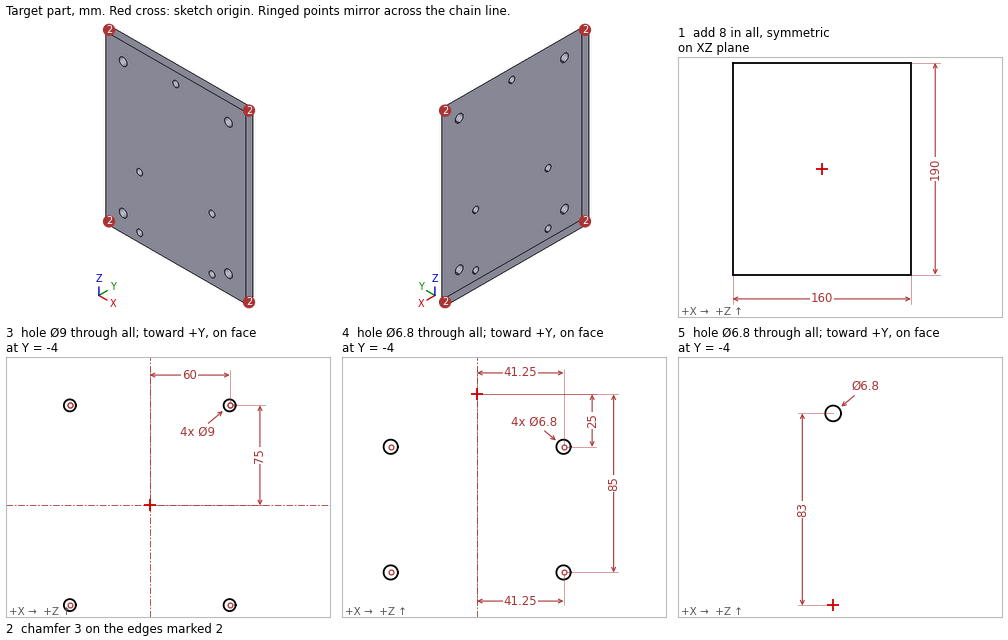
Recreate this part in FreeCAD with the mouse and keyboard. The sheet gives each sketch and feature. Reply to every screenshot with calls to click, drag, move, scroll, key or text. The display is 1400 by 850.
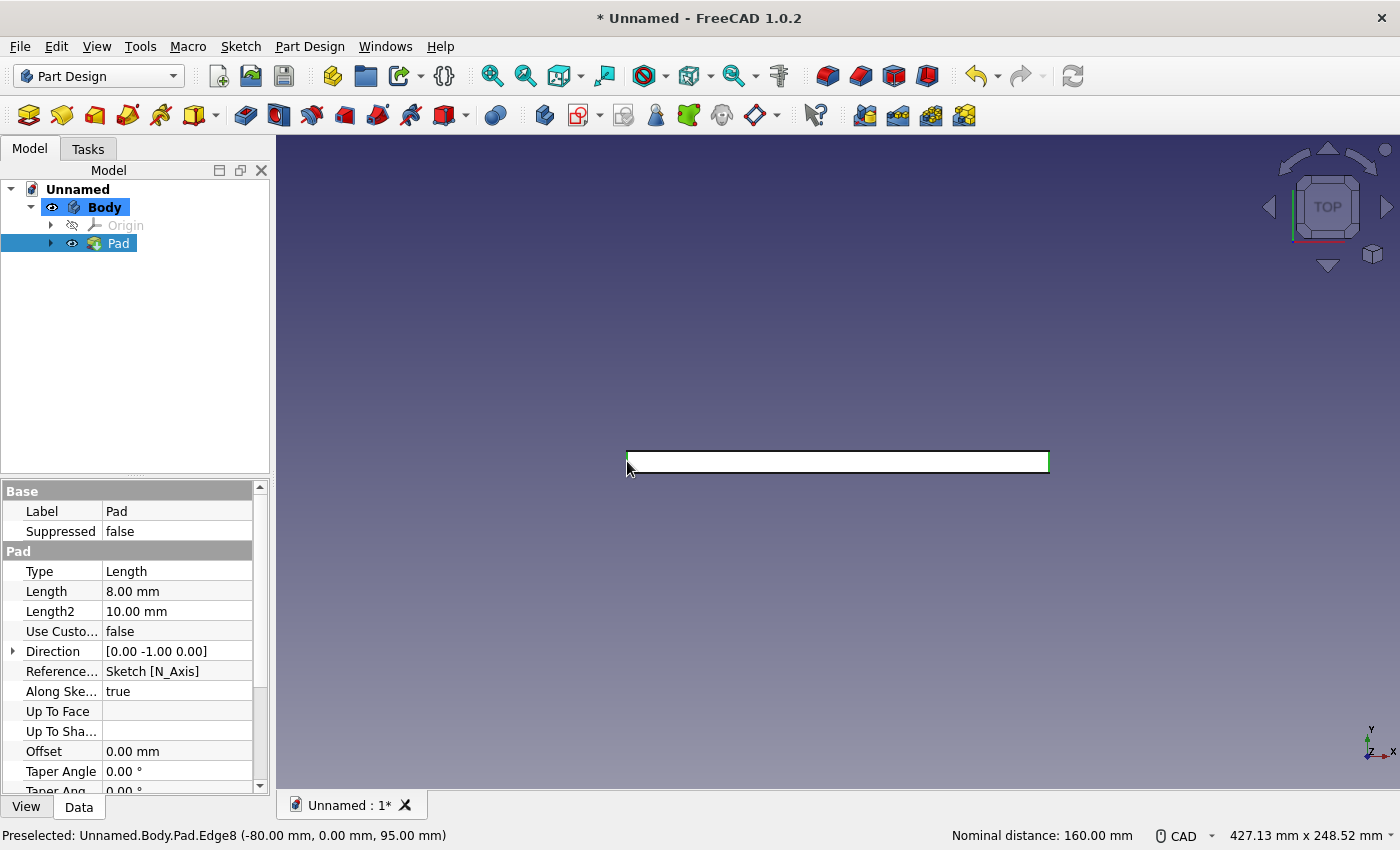
scroll(627, 461, up, 4)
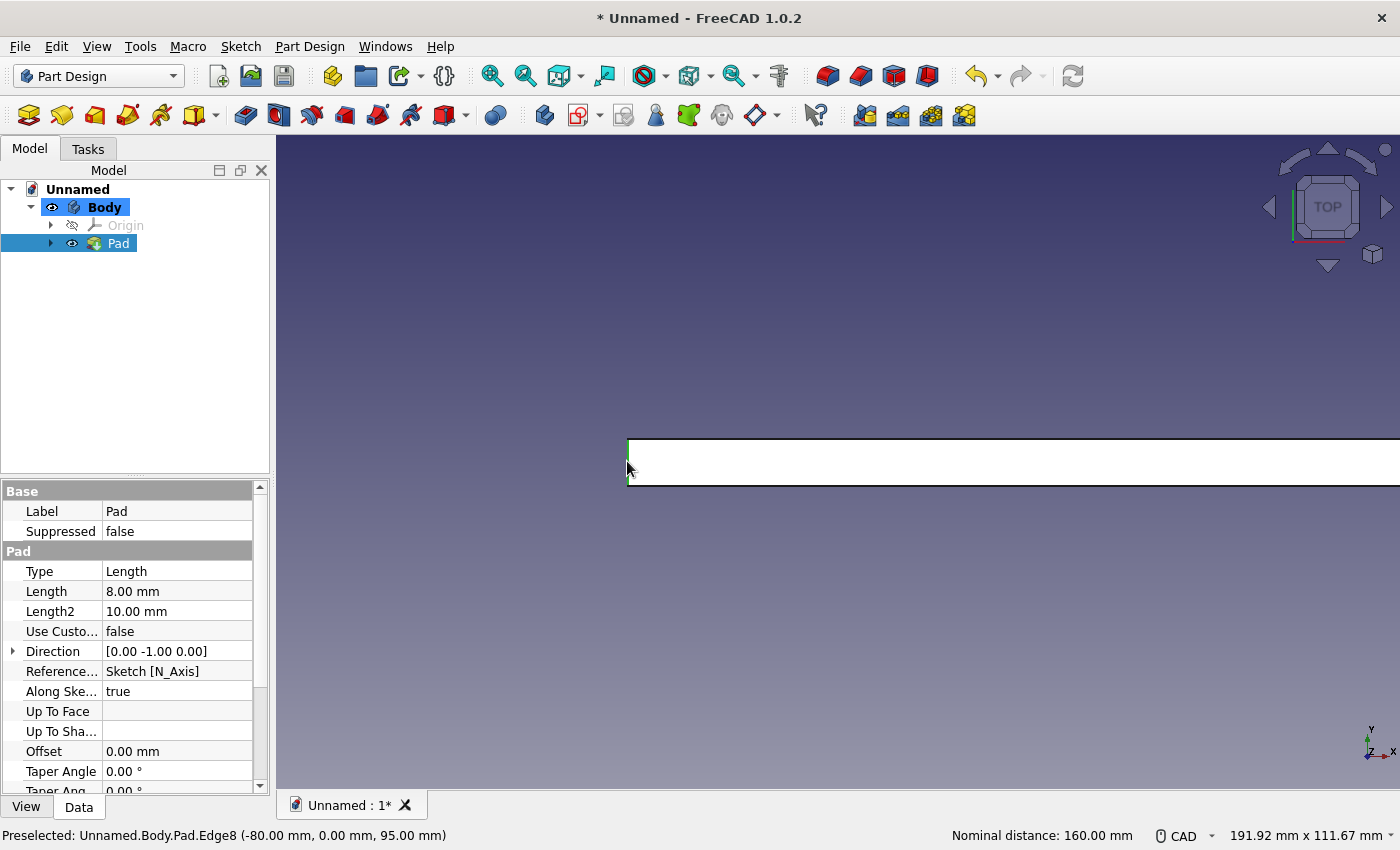
key(v)
key(f)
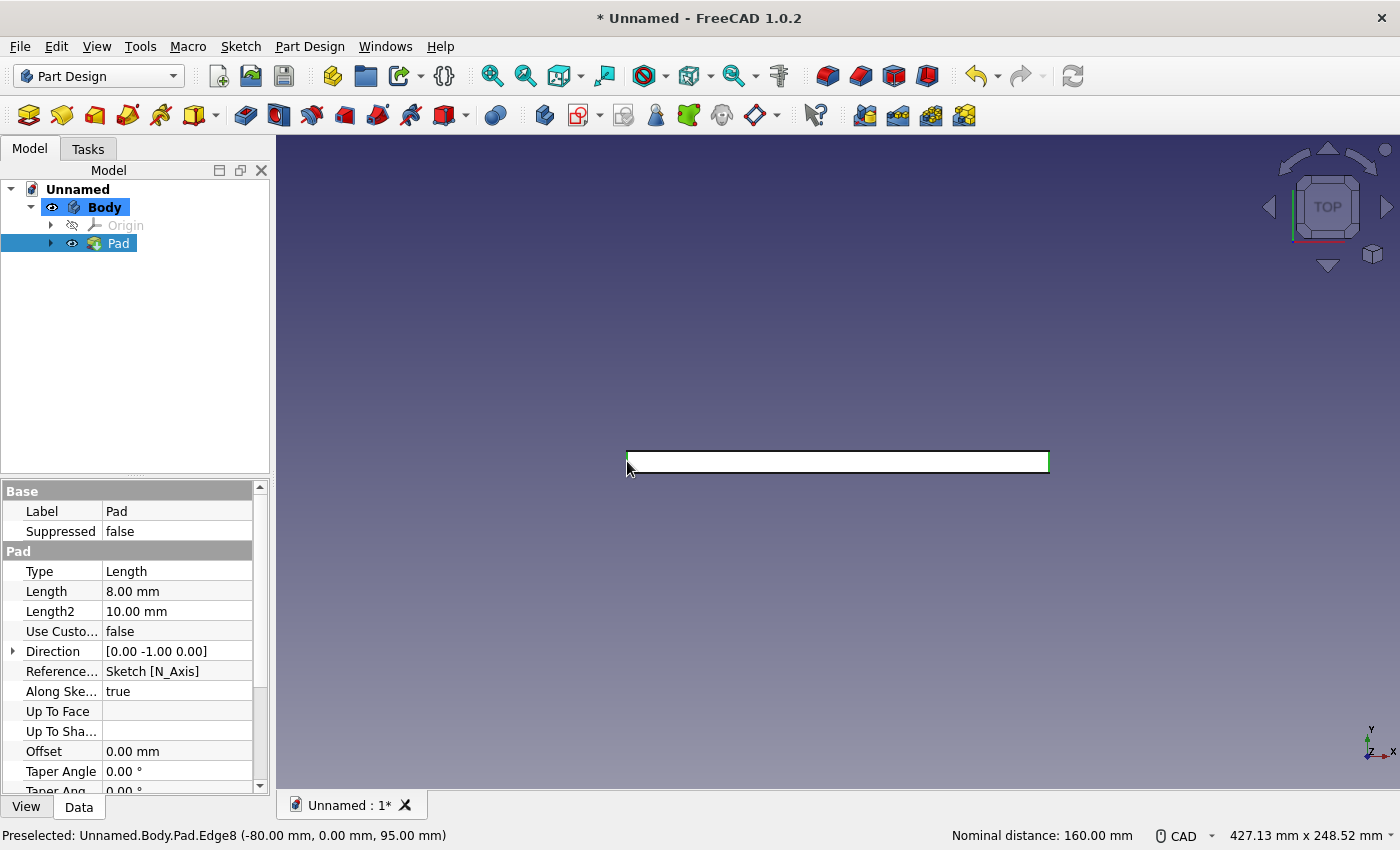
key(1)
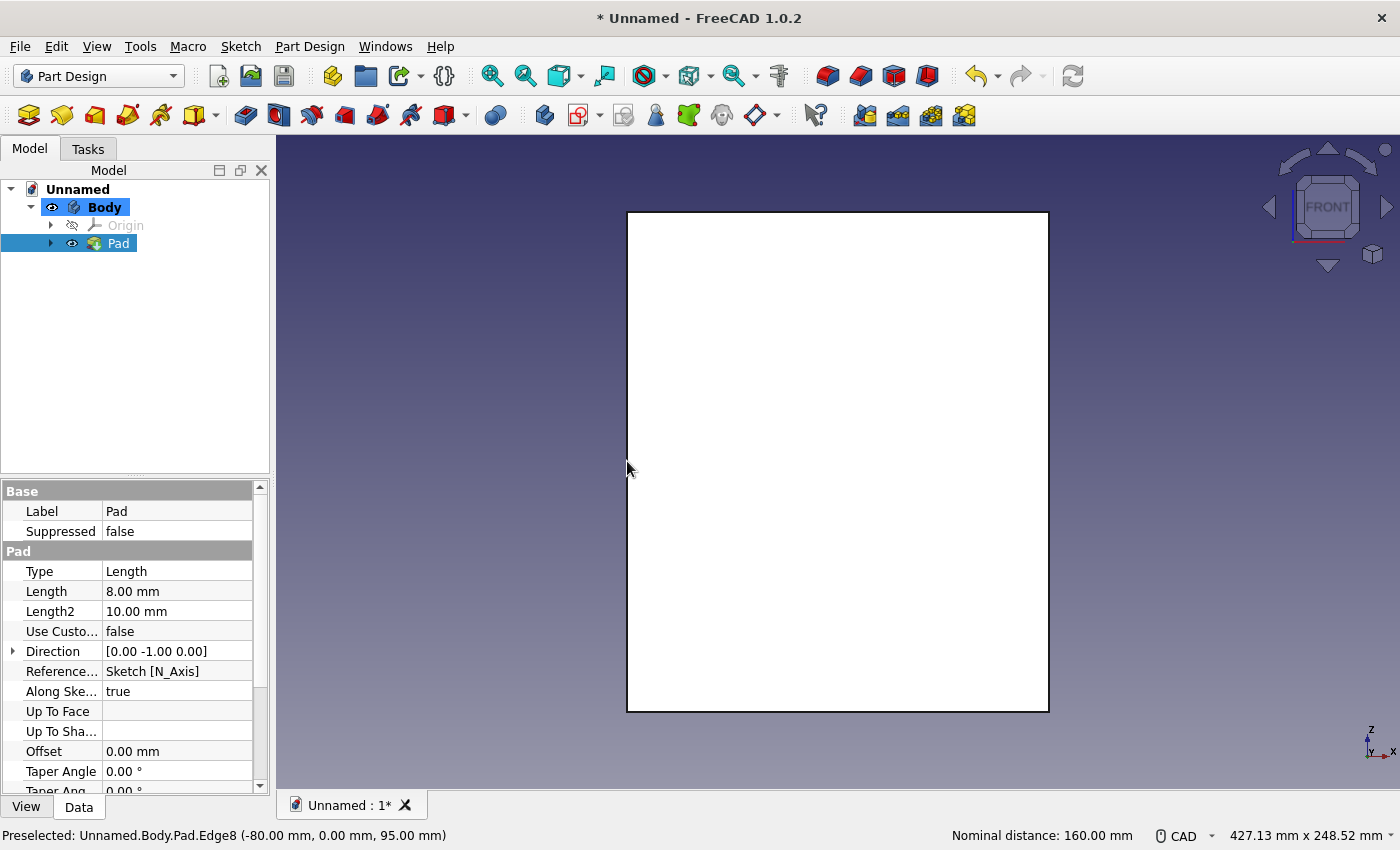
scroll(627, 711, up, 4)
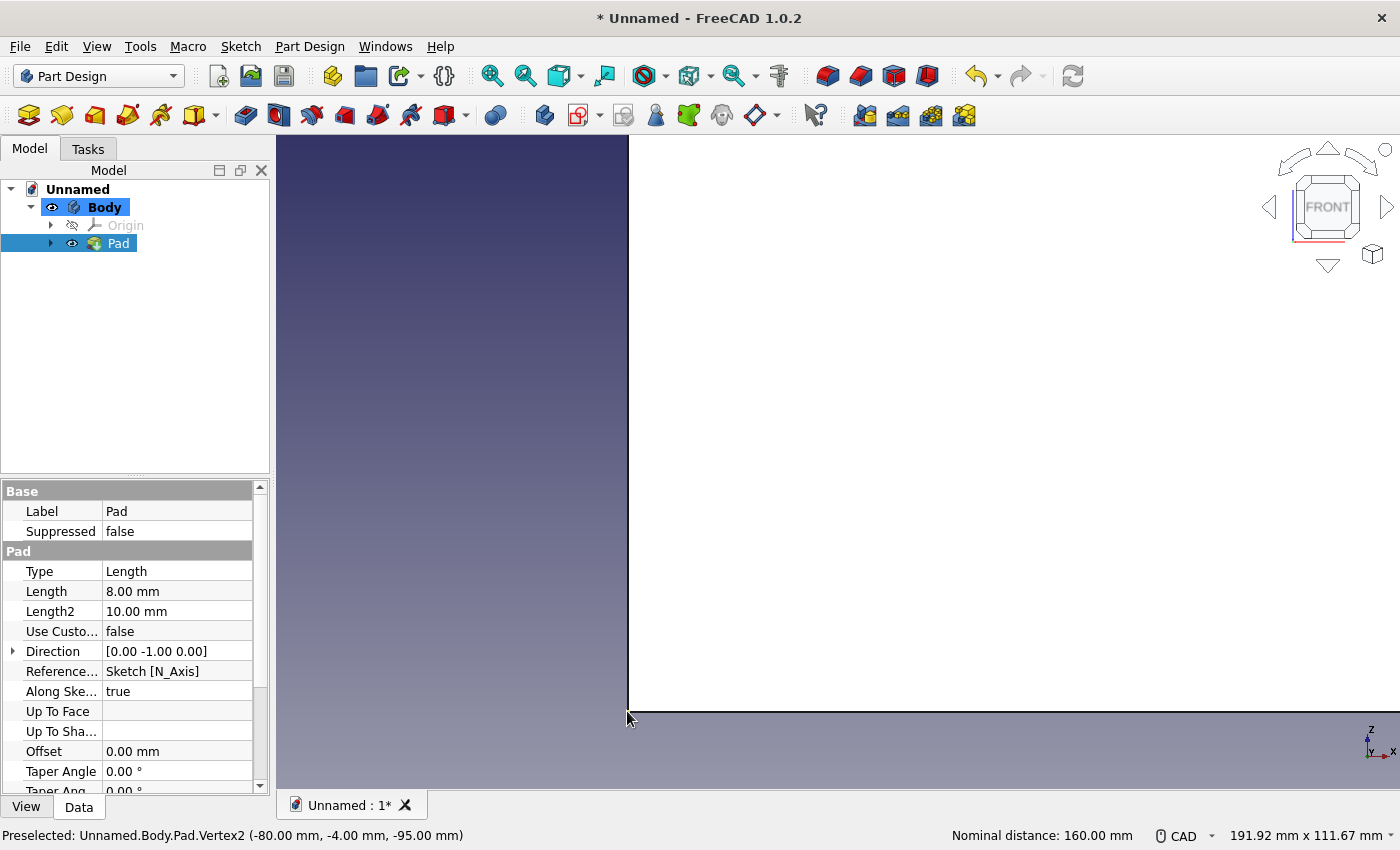
click(493, 76)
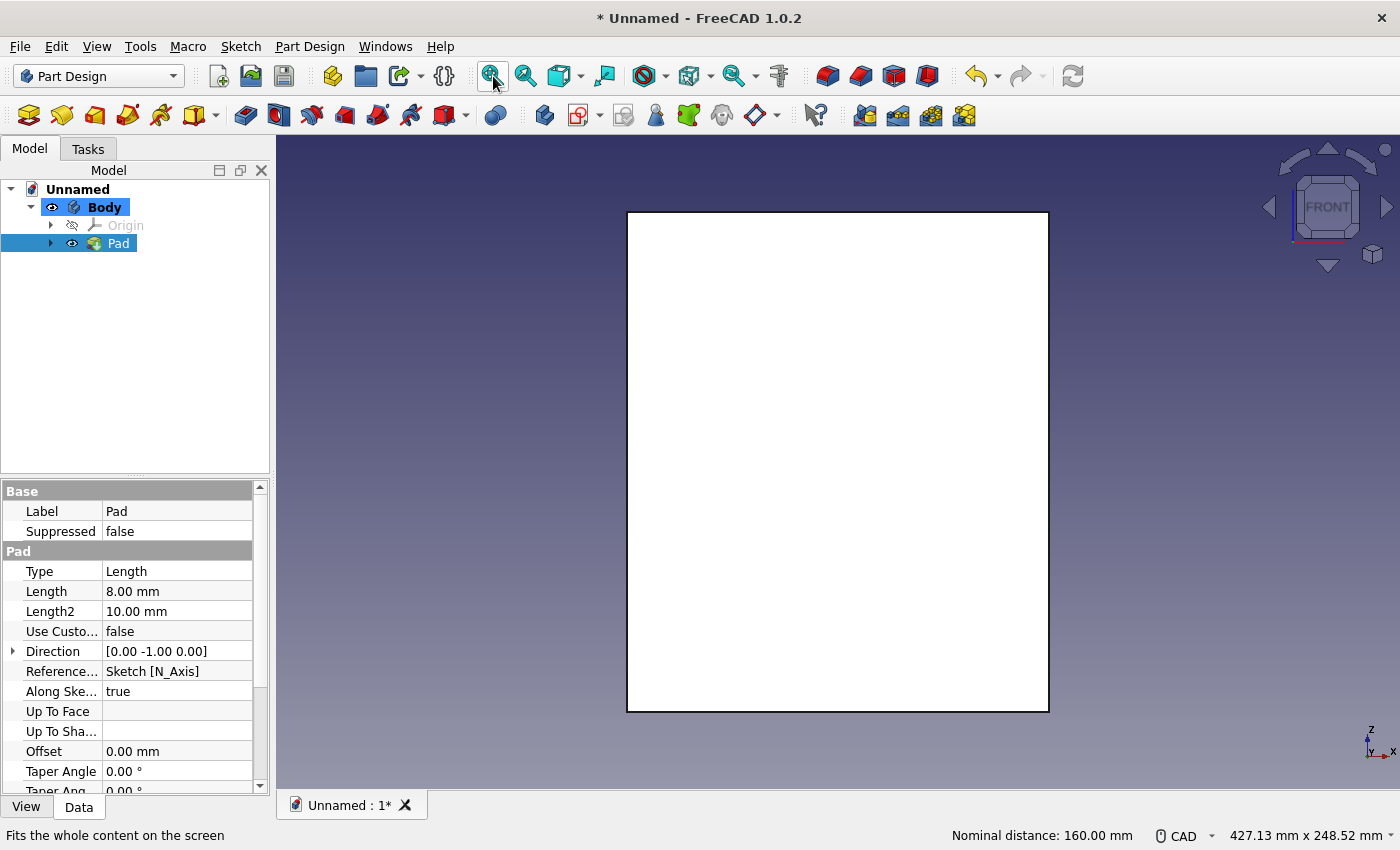
key(3)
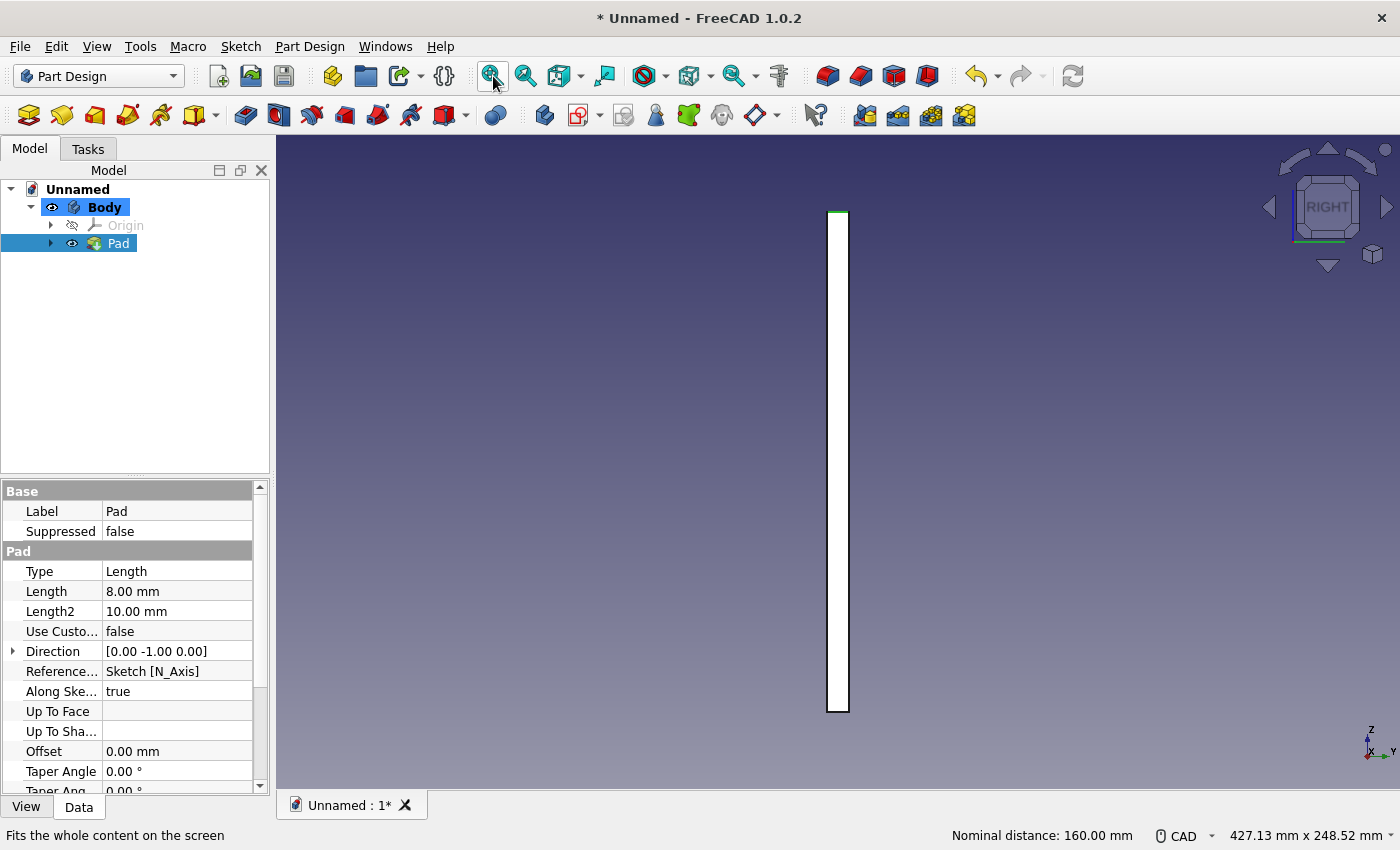
click(838, 711, ctrl)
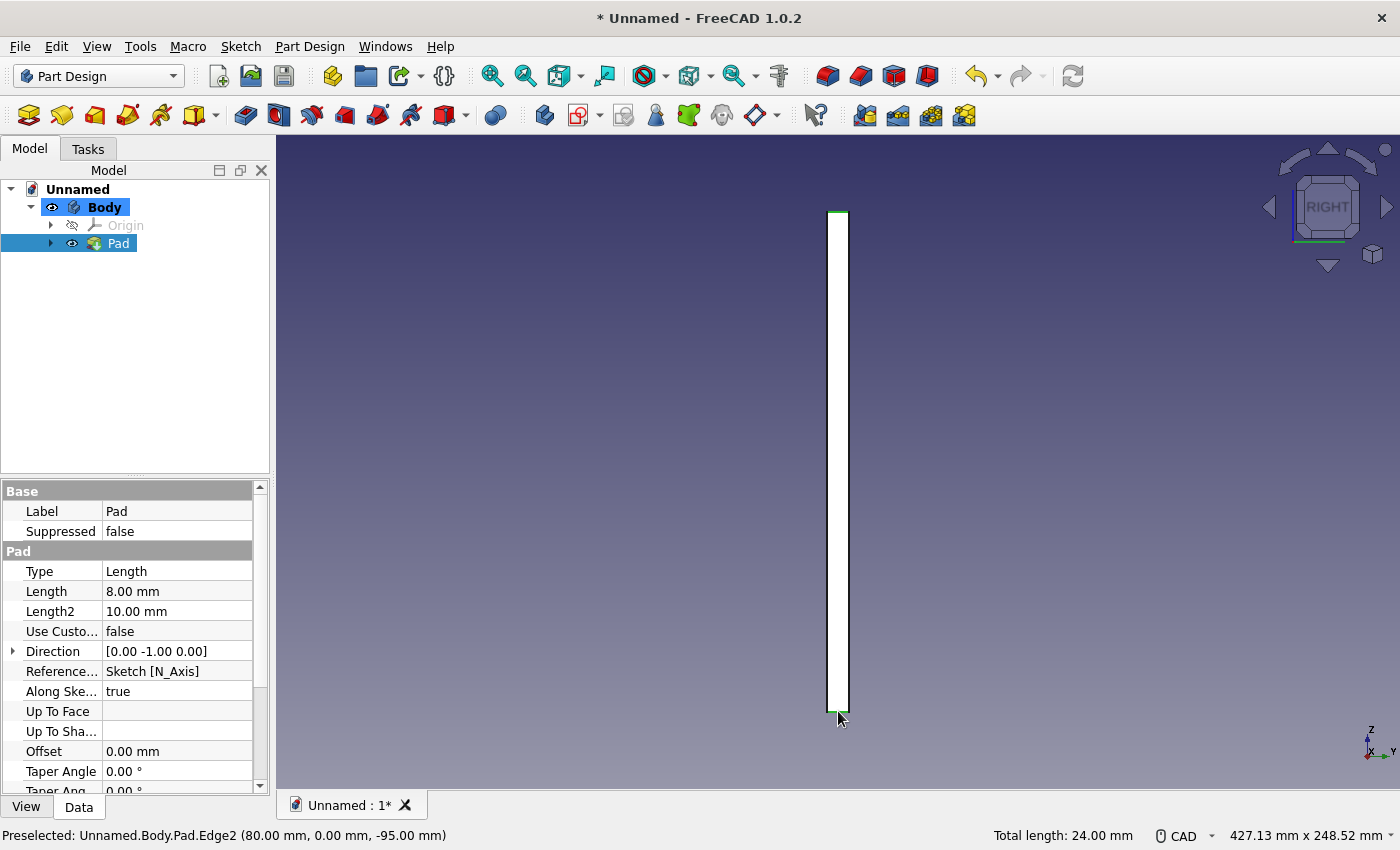
scroll(838, 711, up, 4)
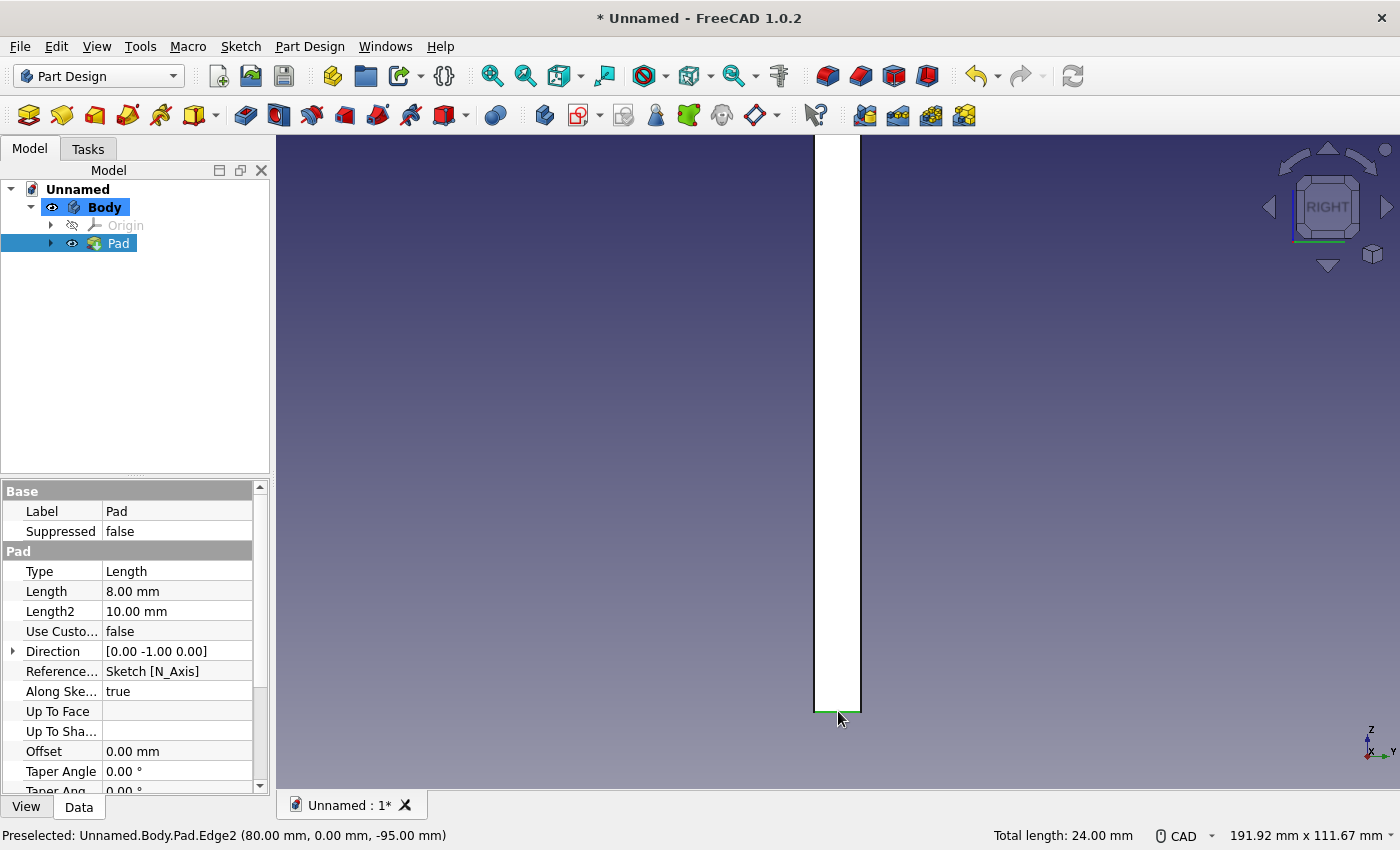
click(493, 76)